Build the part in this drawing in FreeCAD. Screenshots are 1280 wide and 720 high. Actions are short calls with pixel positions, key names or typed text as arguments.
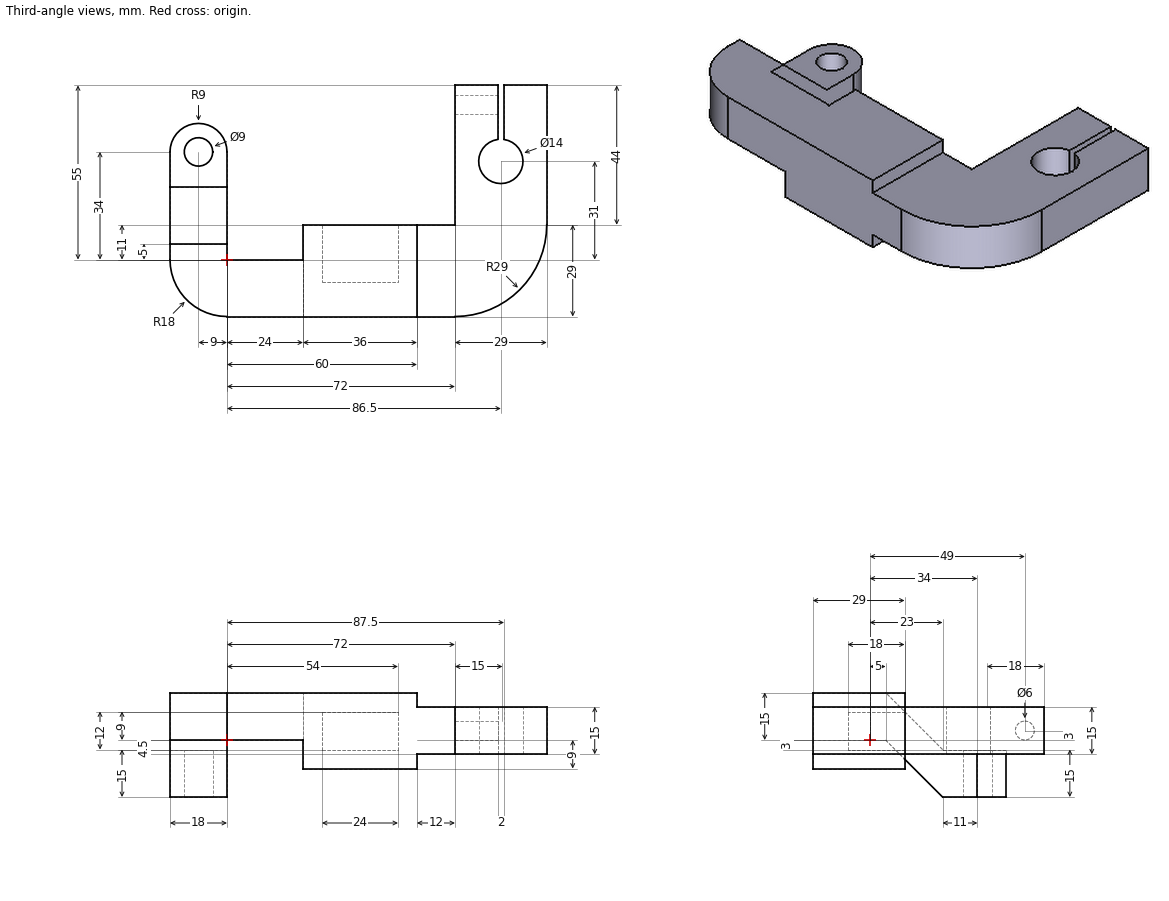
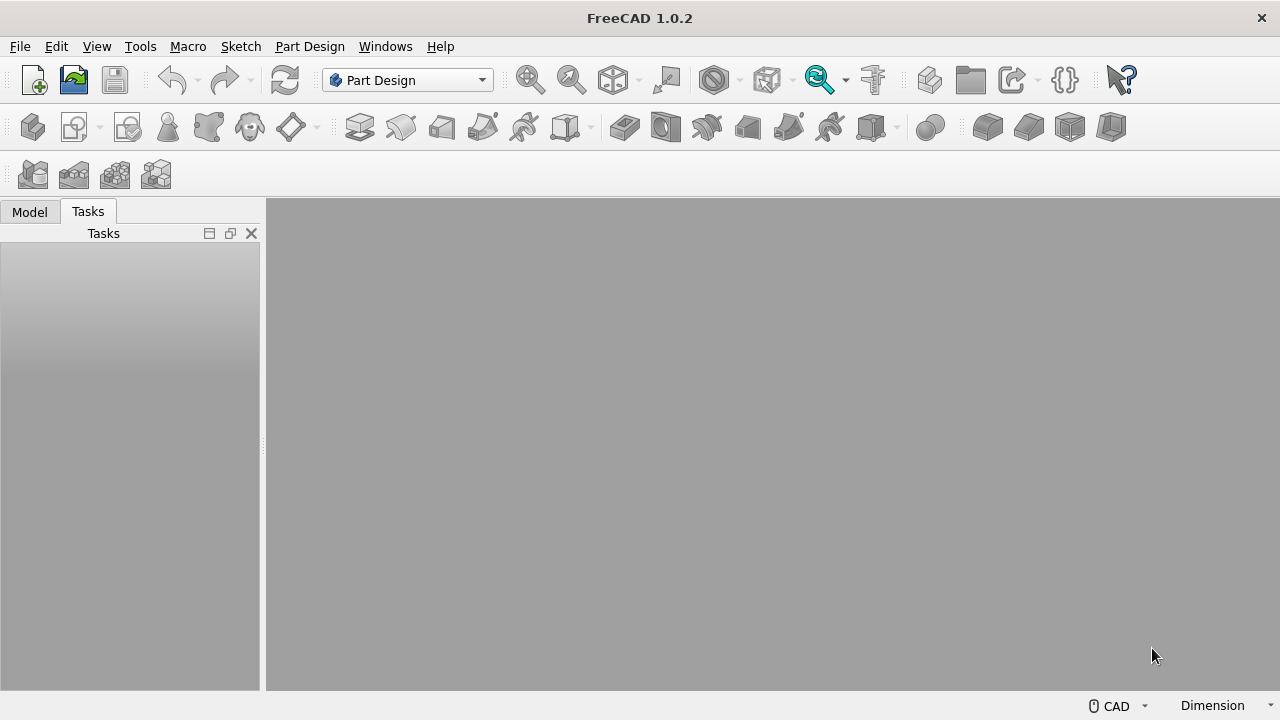
click(33, 80)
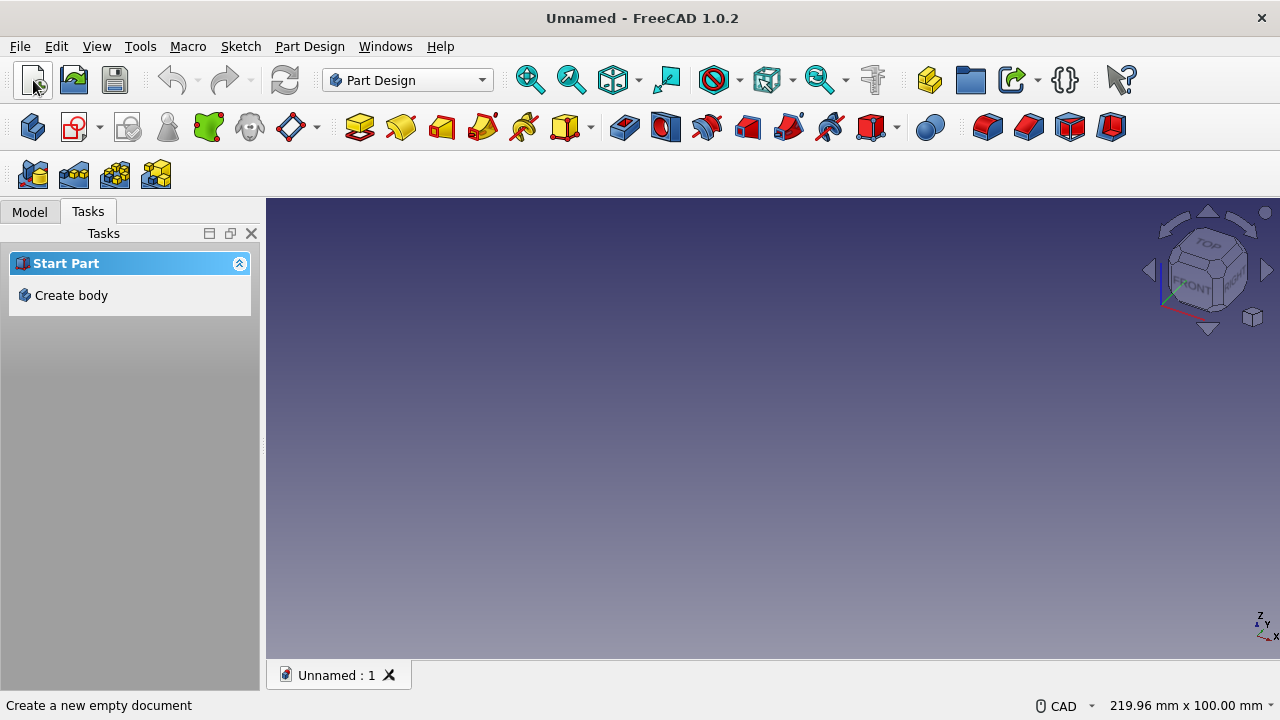
click(74, 128)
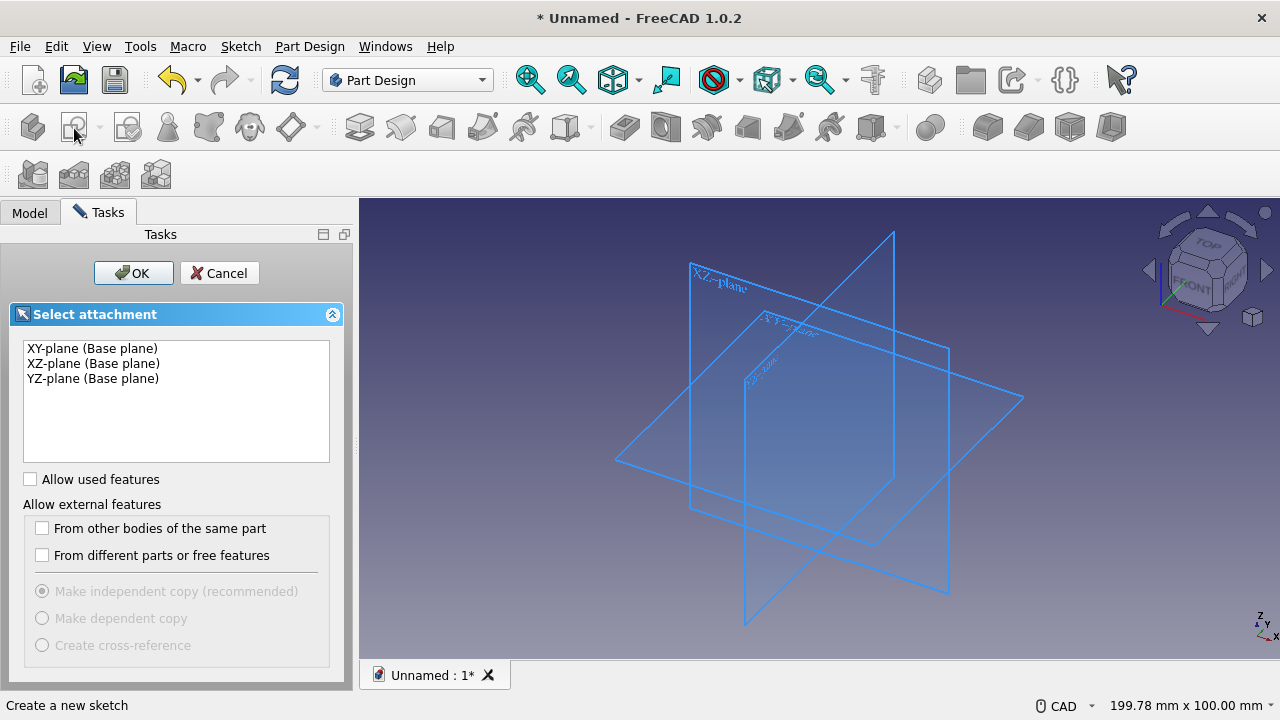
click(84, 348)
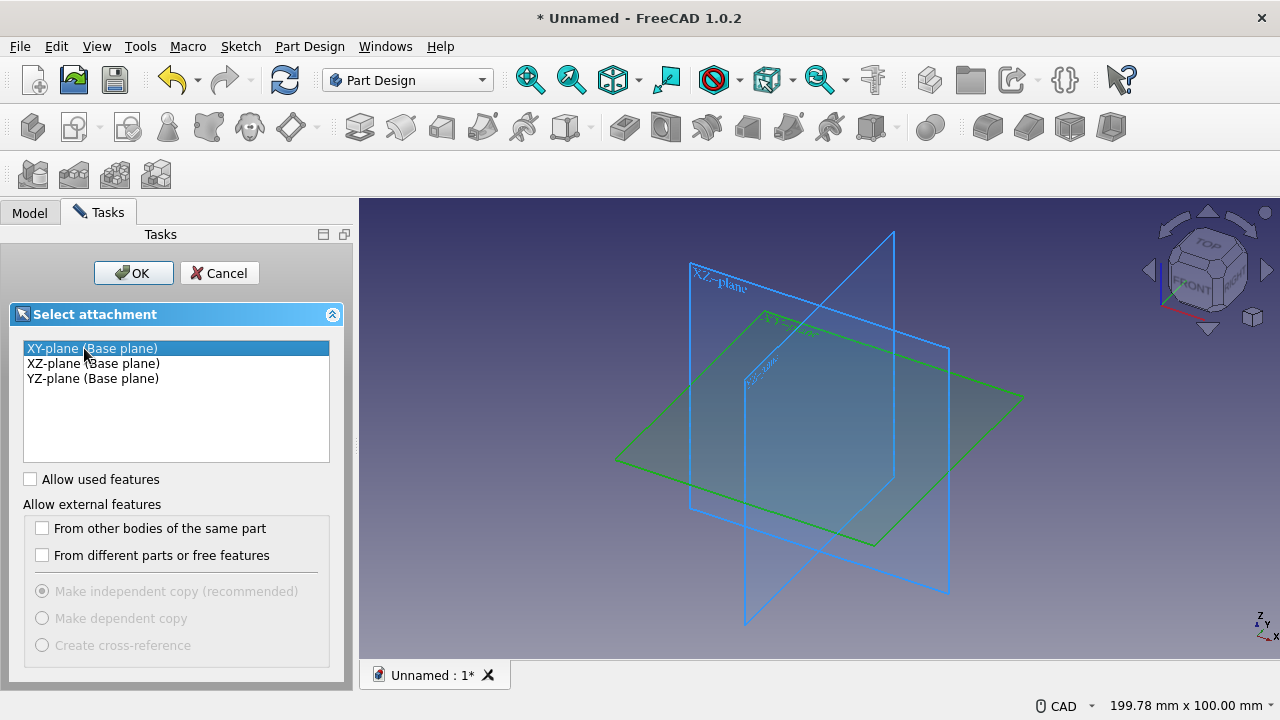
click(134, 273)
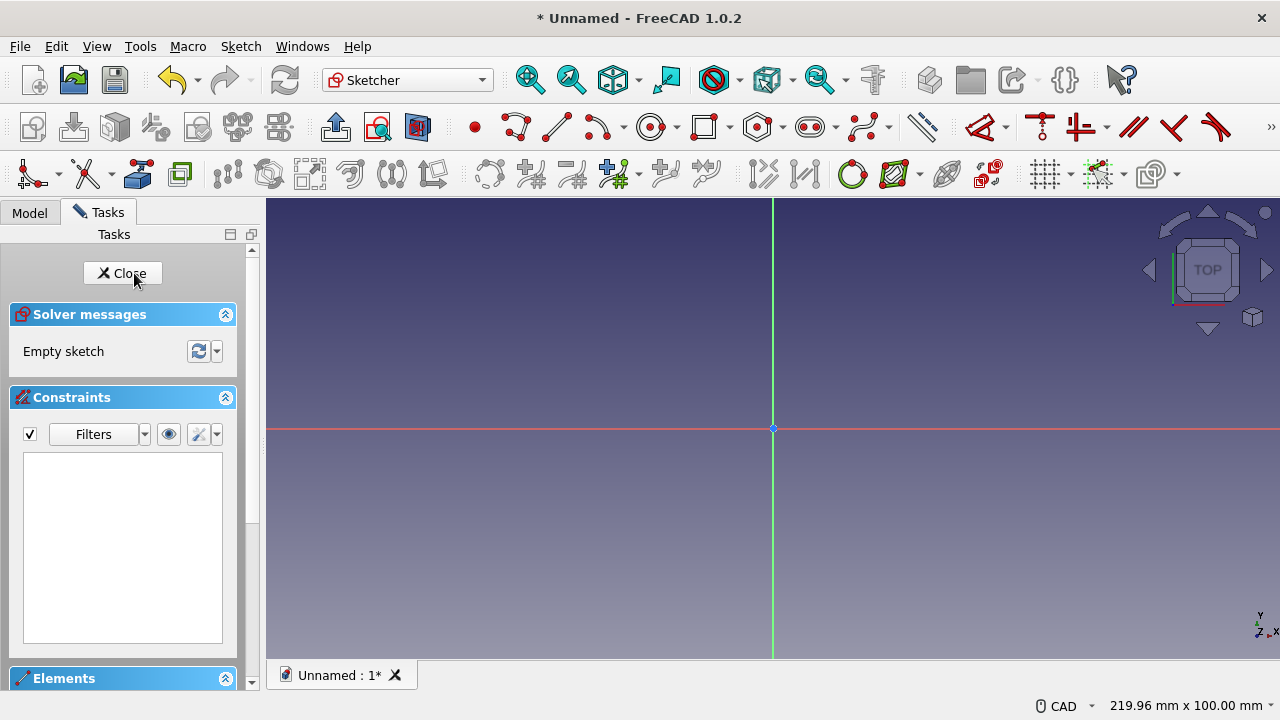
scroll(1115, 477, up, 2)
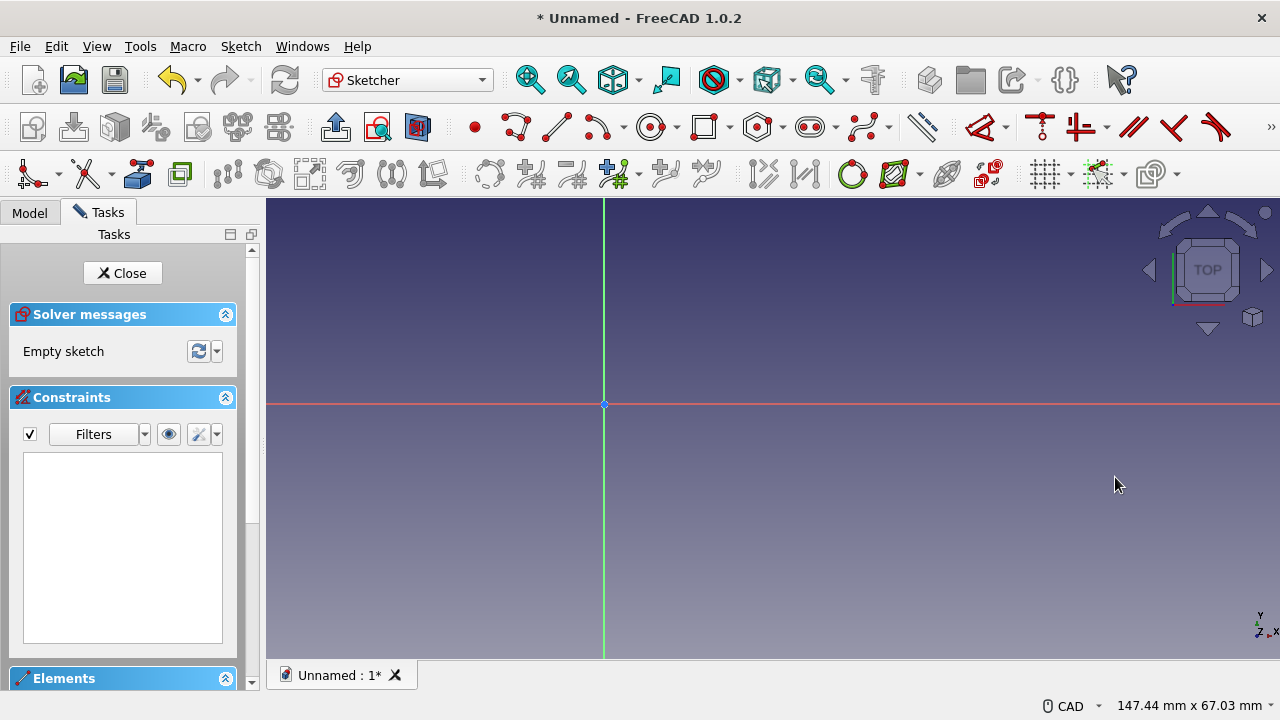
click(516, 128)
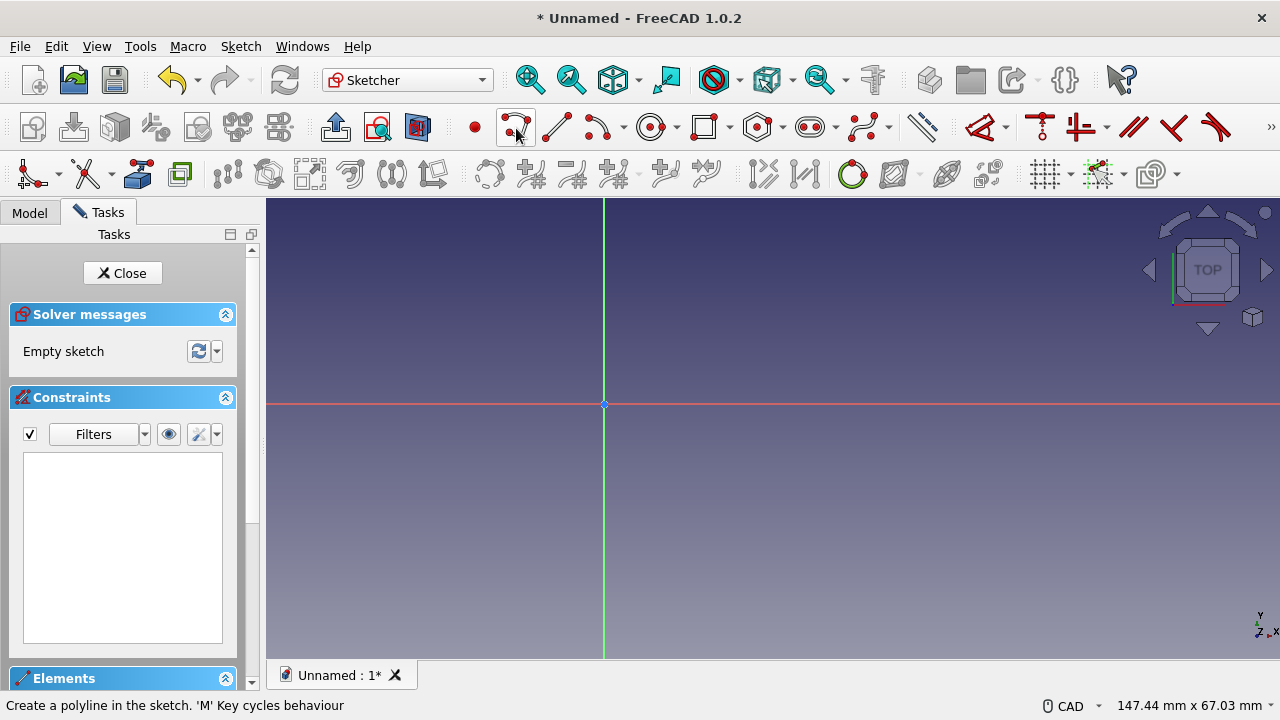
click(604, 528)
click(1017, 528)
click(1017, 329)
click(769, 329)
click(769, 404)
click(604, 404)
click(613, 370)
click(481, 370)
click(481, 404)
right_click(481, 404)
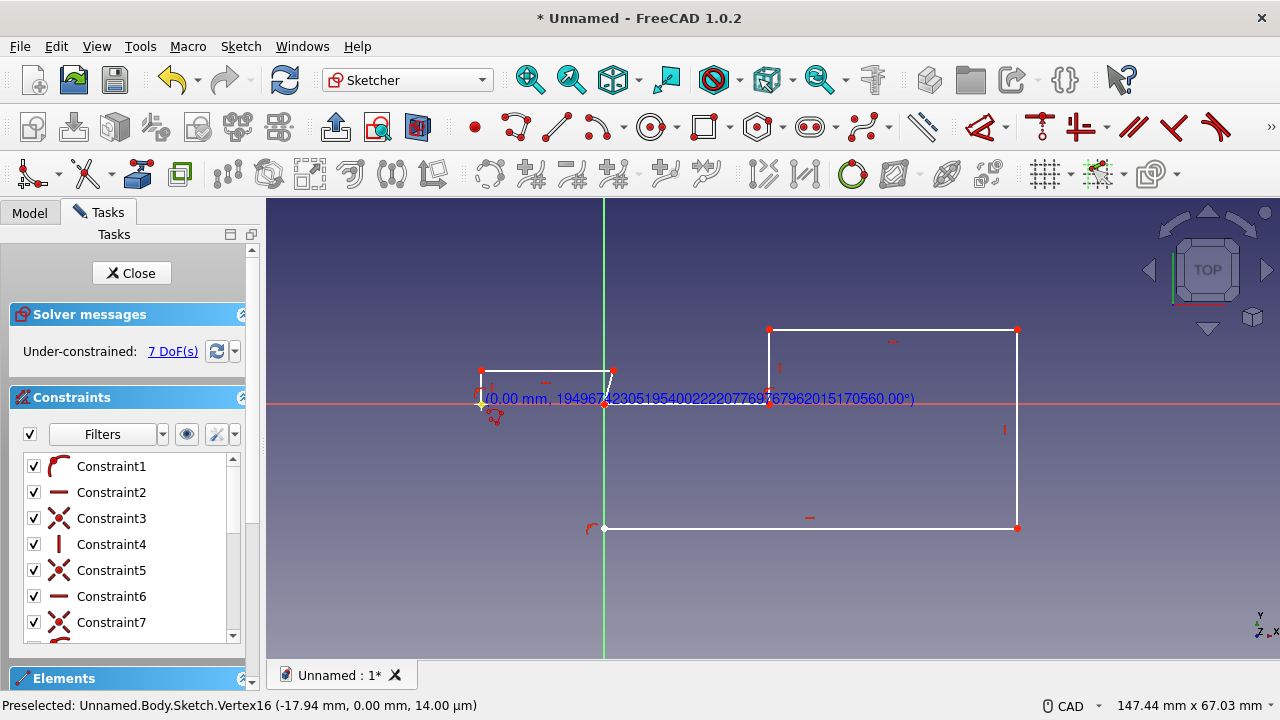
click(624, 128)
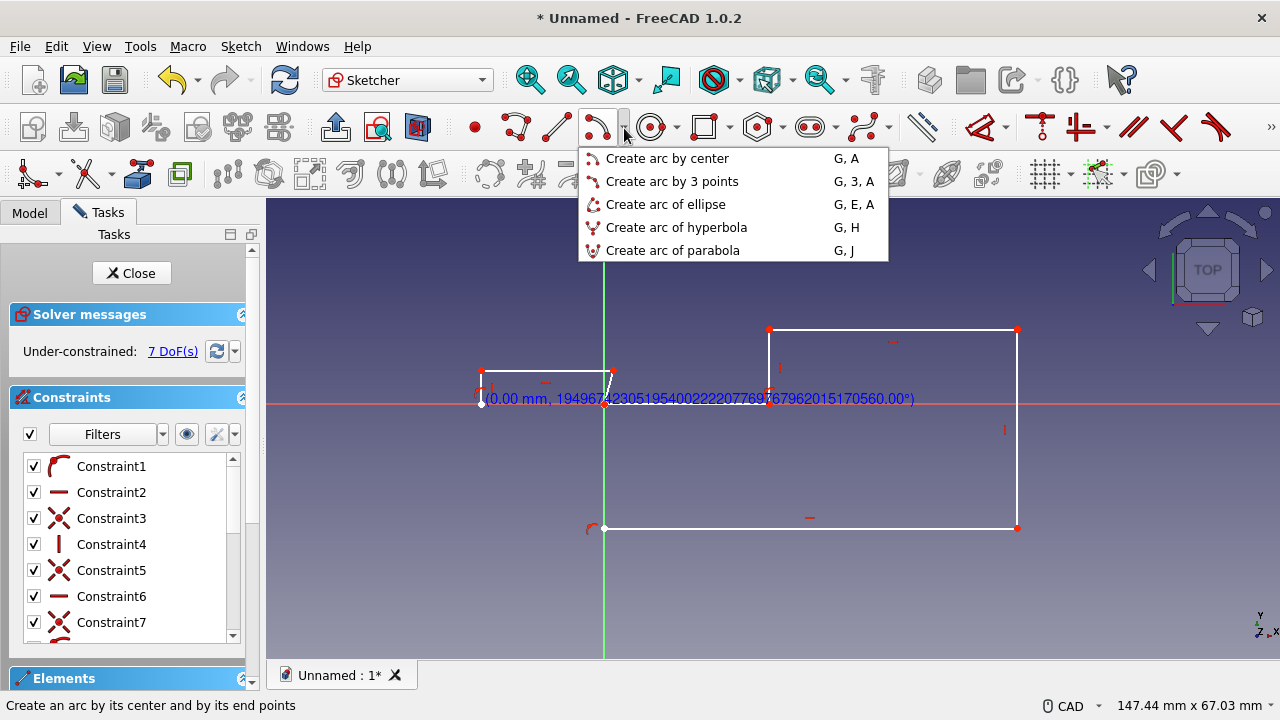
click(734, 182)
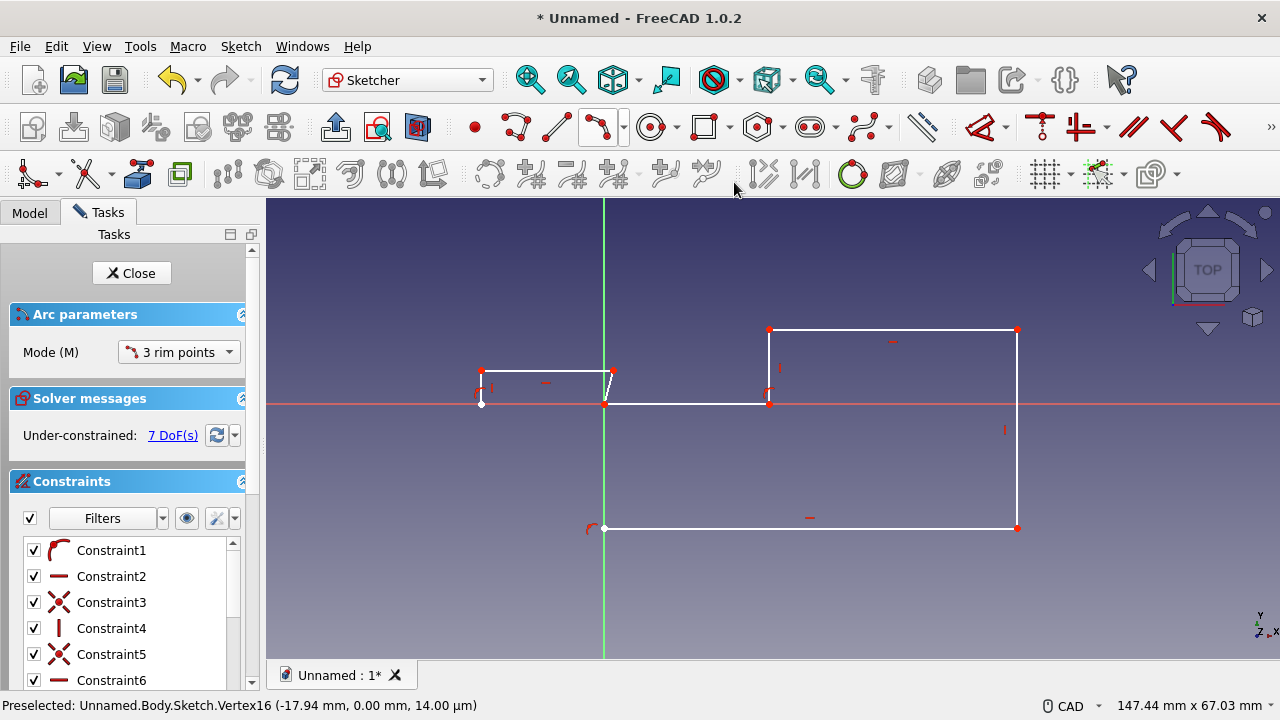
click(481, 404)
click(604, 529)
click(517, 492)
key(Escape)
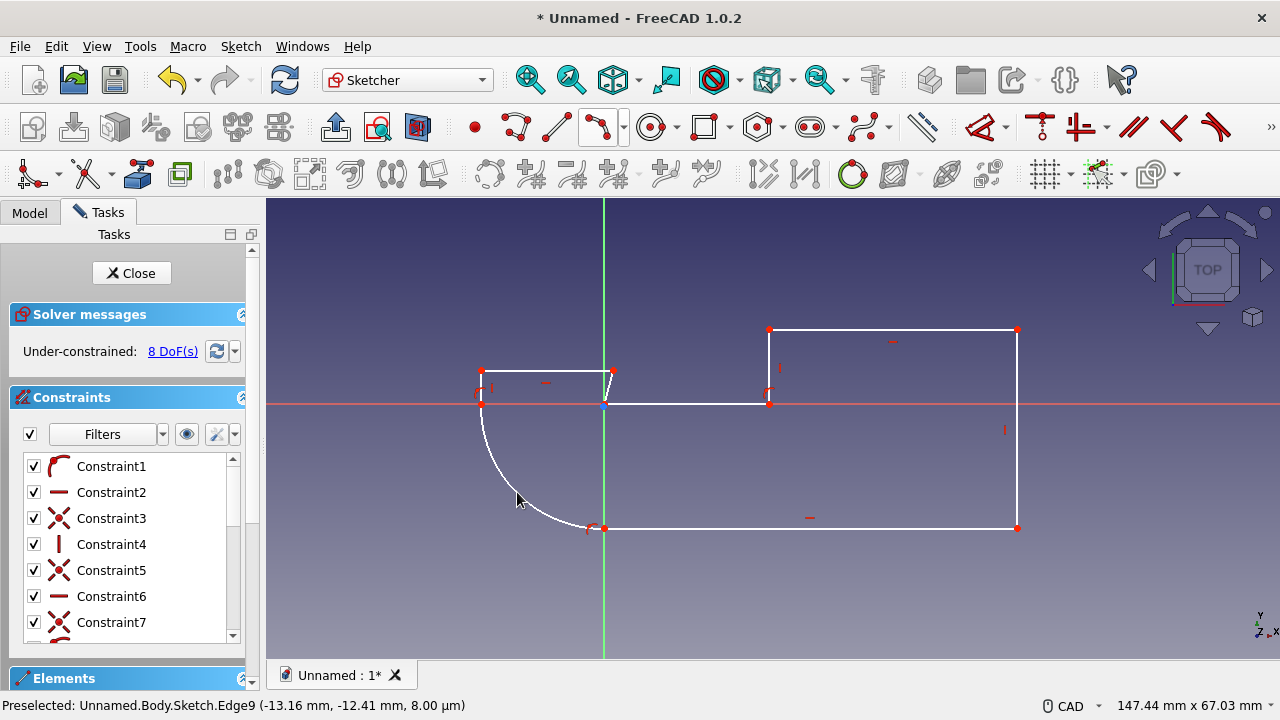
click(728, 529)